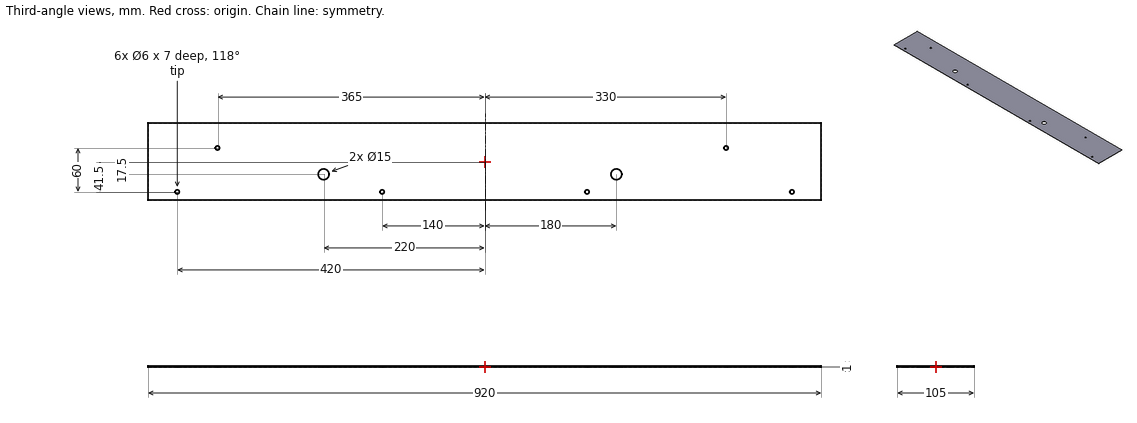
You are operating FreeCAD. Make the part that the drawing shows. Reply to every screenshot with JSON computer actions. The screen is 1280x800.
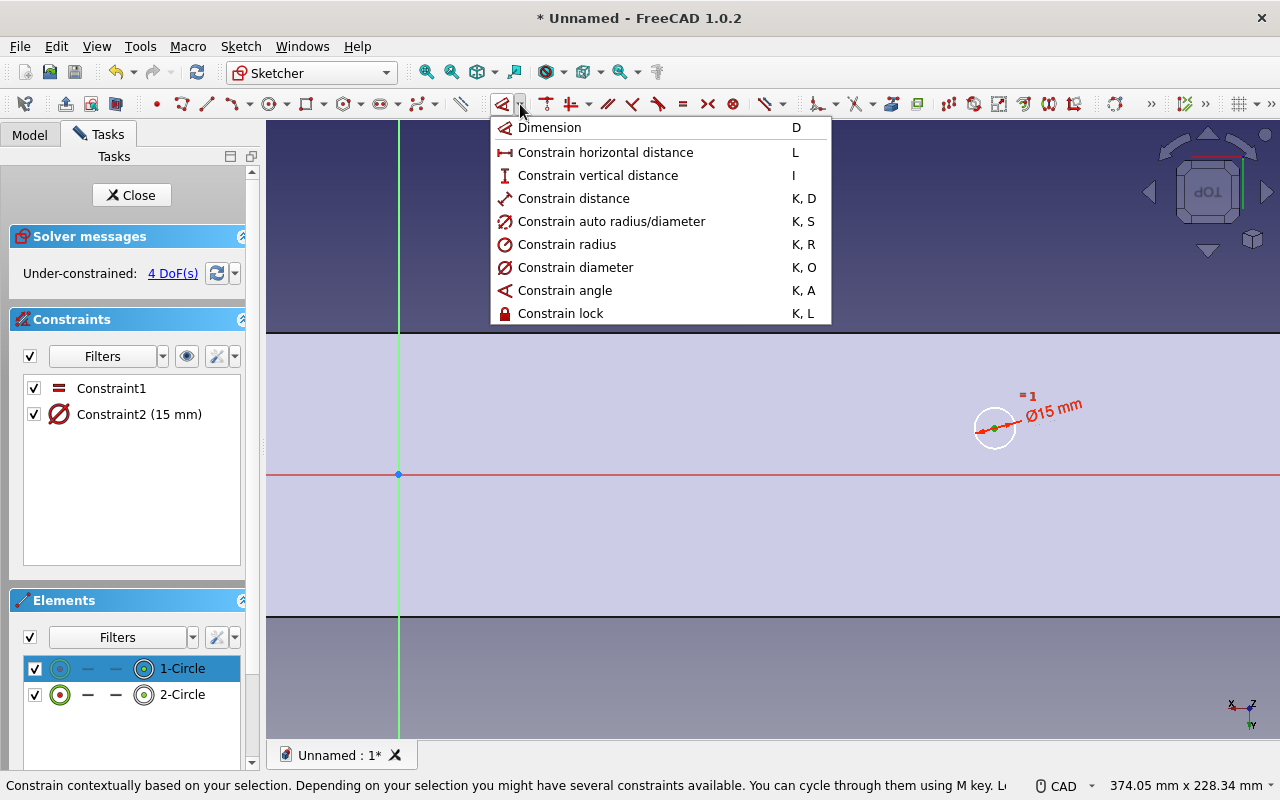
{"action": "left_click", "coordinate": [661, 152]}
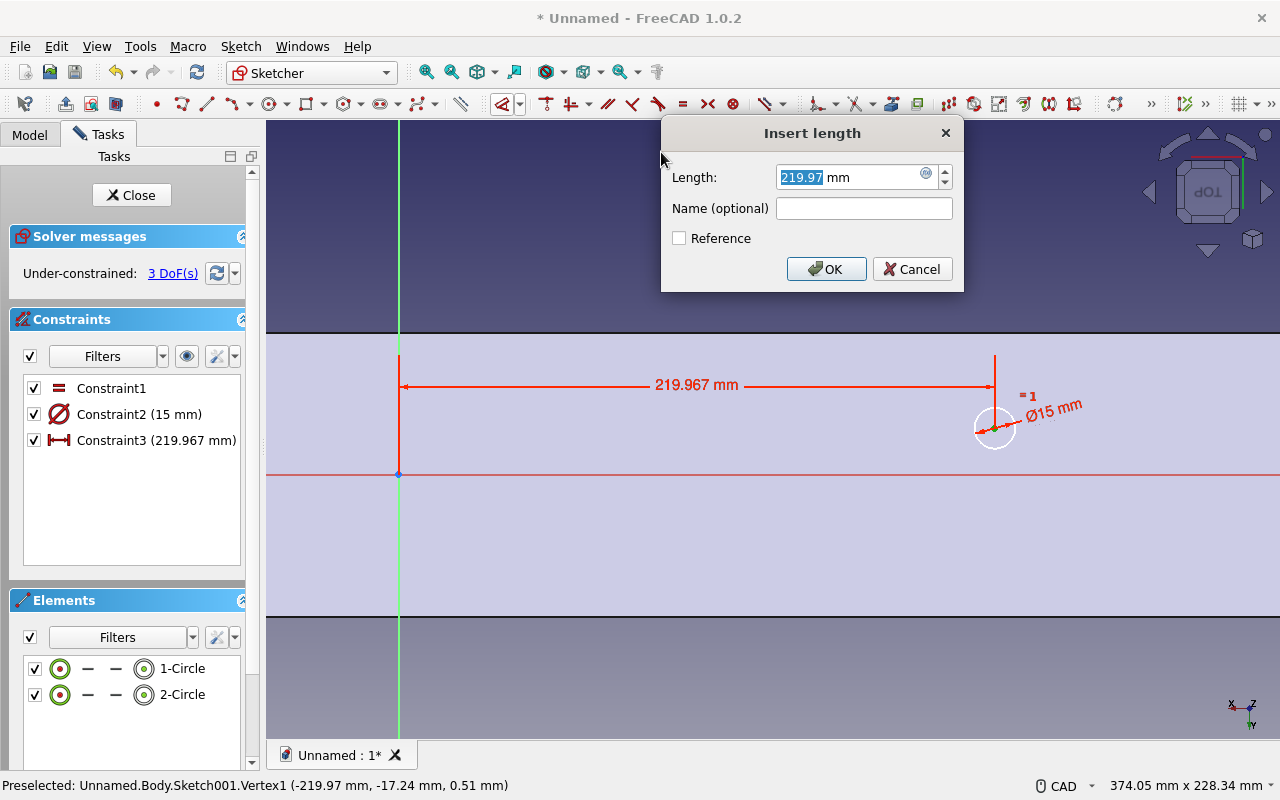
{"action": "type", "text": "220"}
{"action": "key", "text": "Return"}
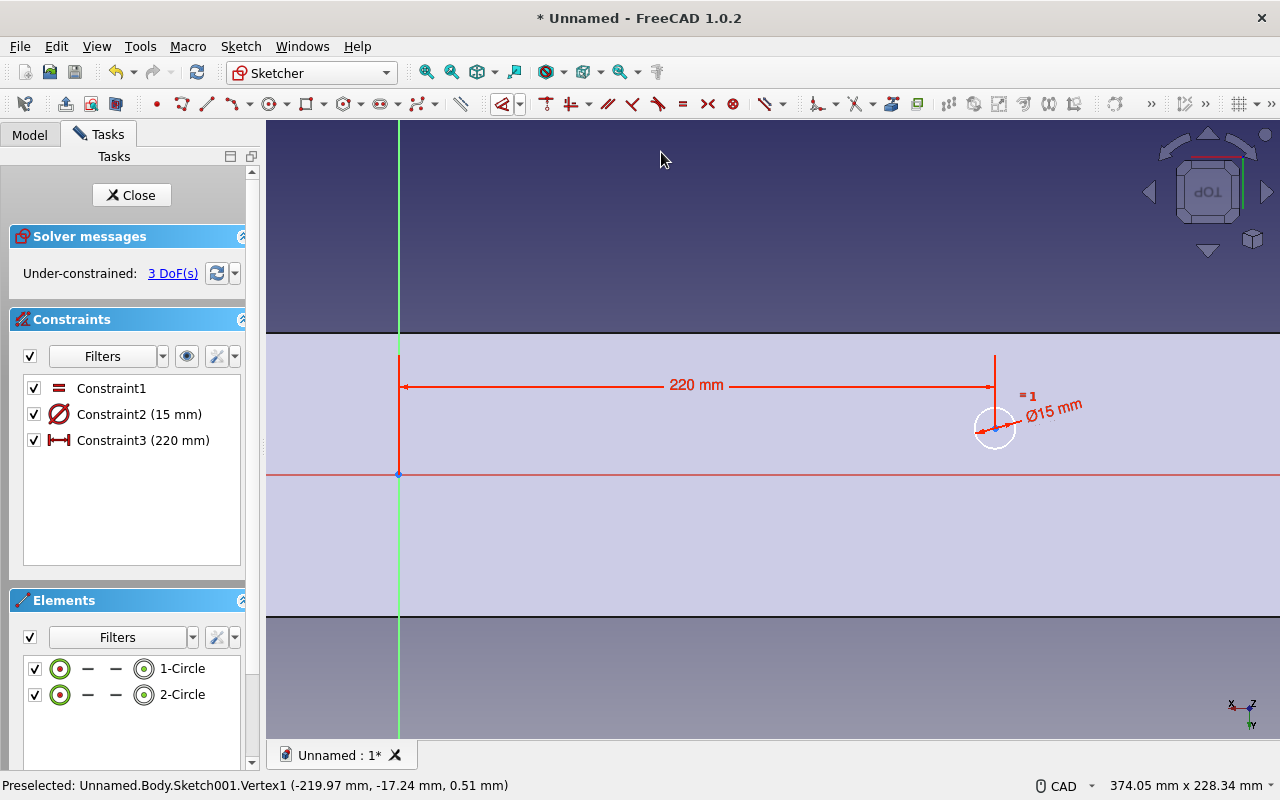
{"action": "scroll", "coordinate": [1011, 415], "scroll_direction": "down", "scroll_amount": 3}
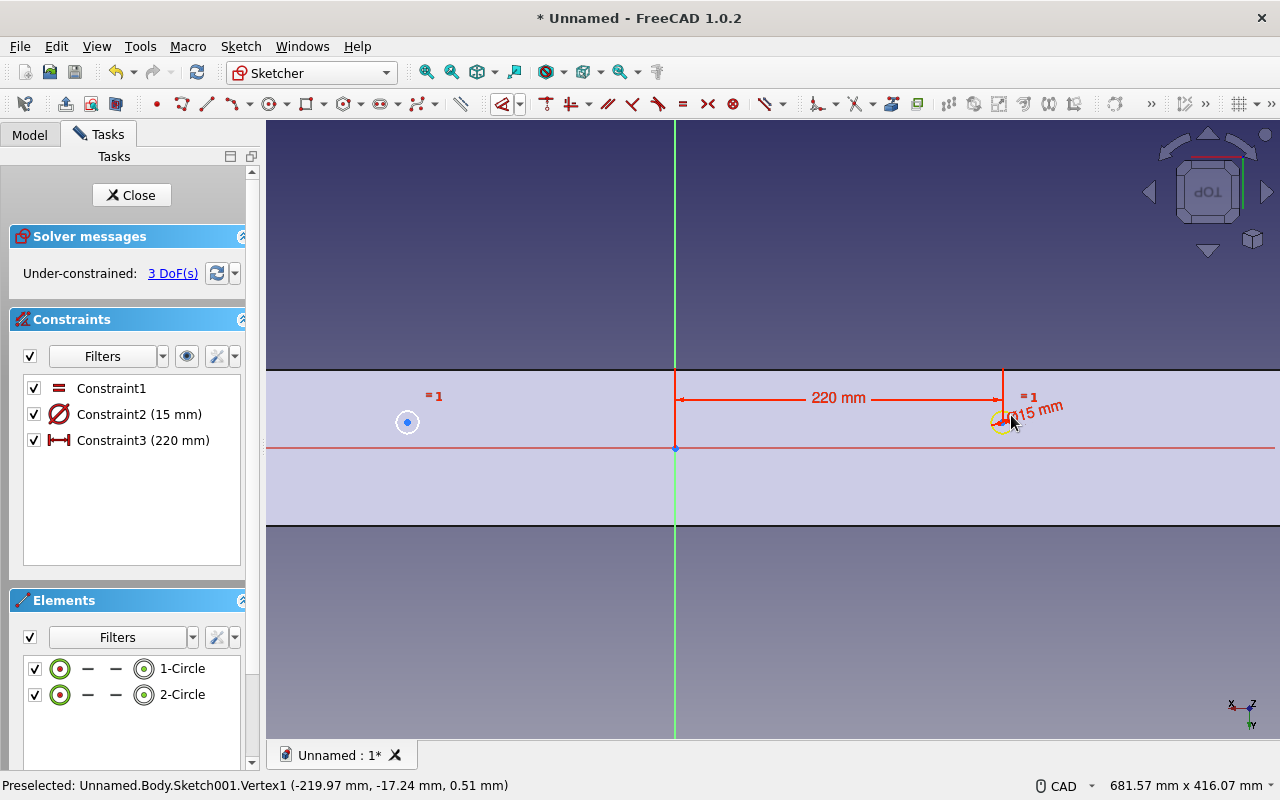
{"action": "left_click", "coordinate": [408, 422]}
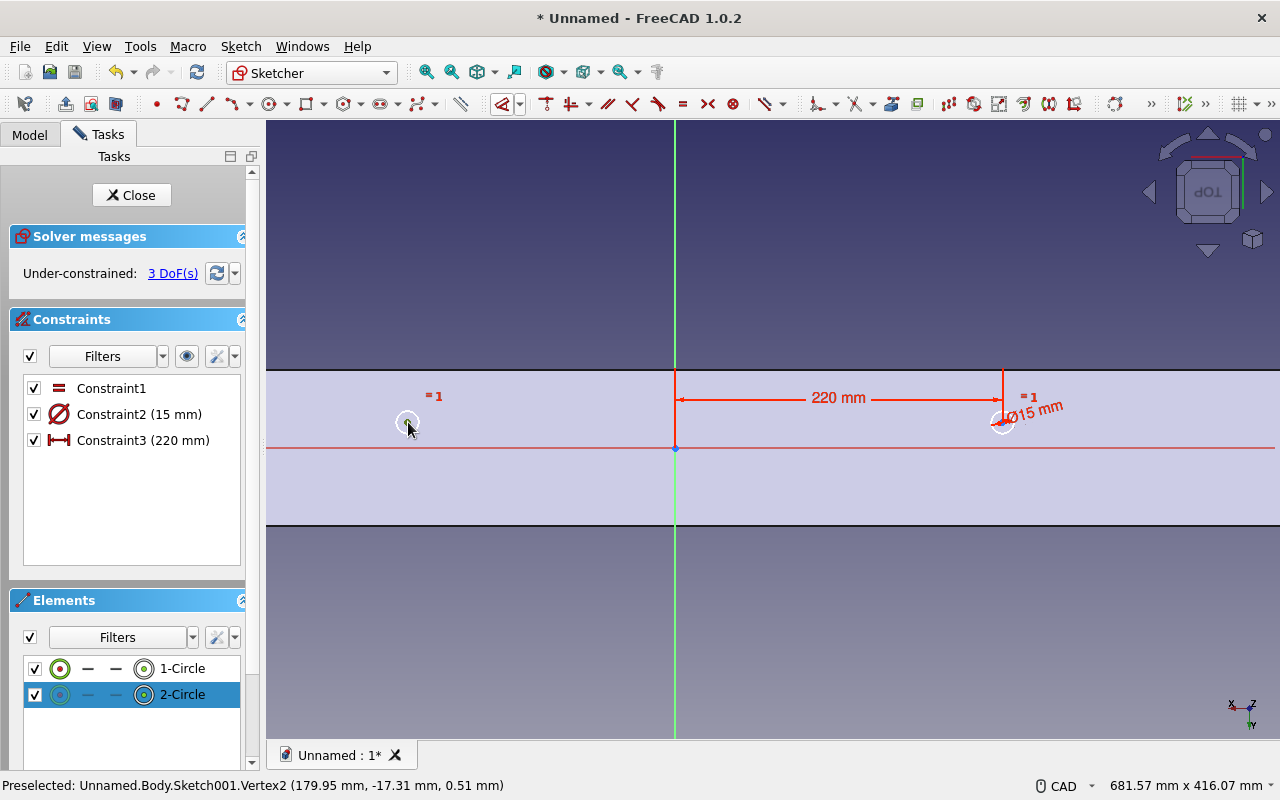
{"action": "left_click", "coordinate": [520, 104]}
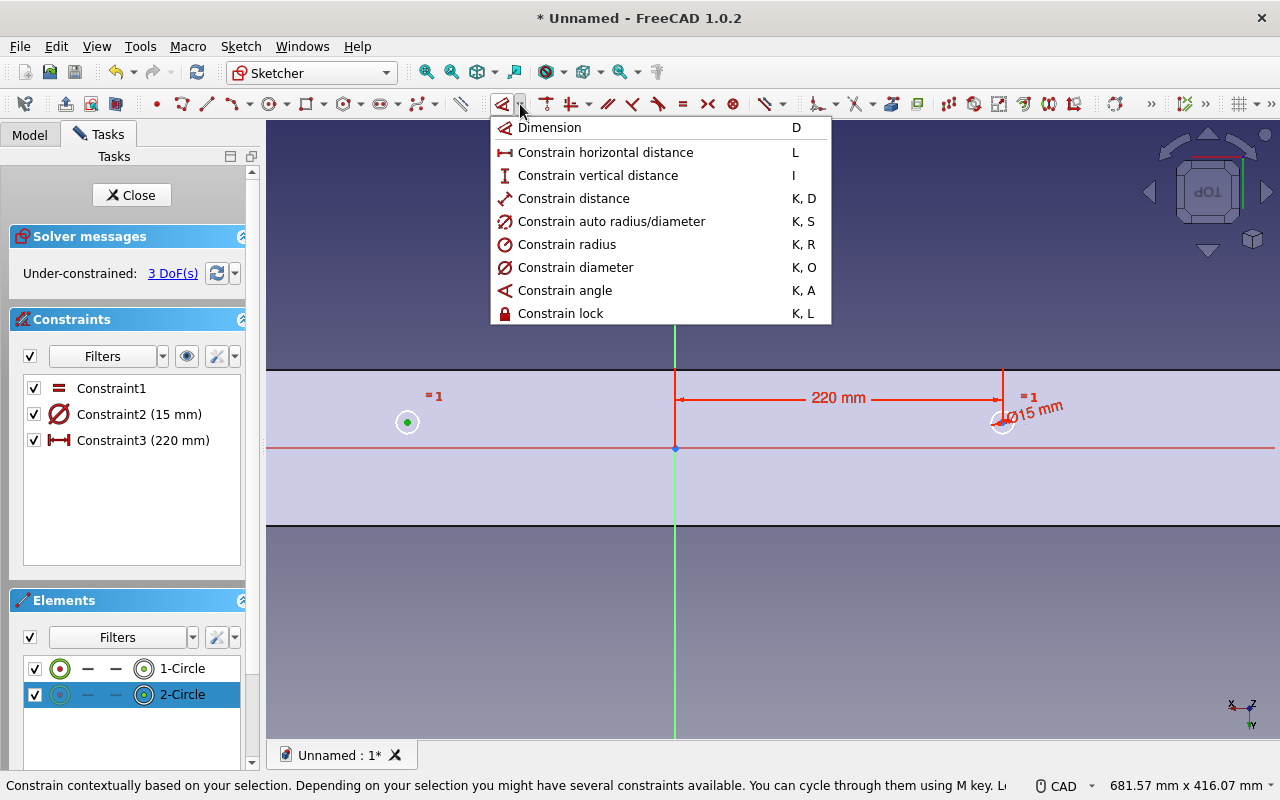
{"action": "left_click", "coordinate": [661, 152]}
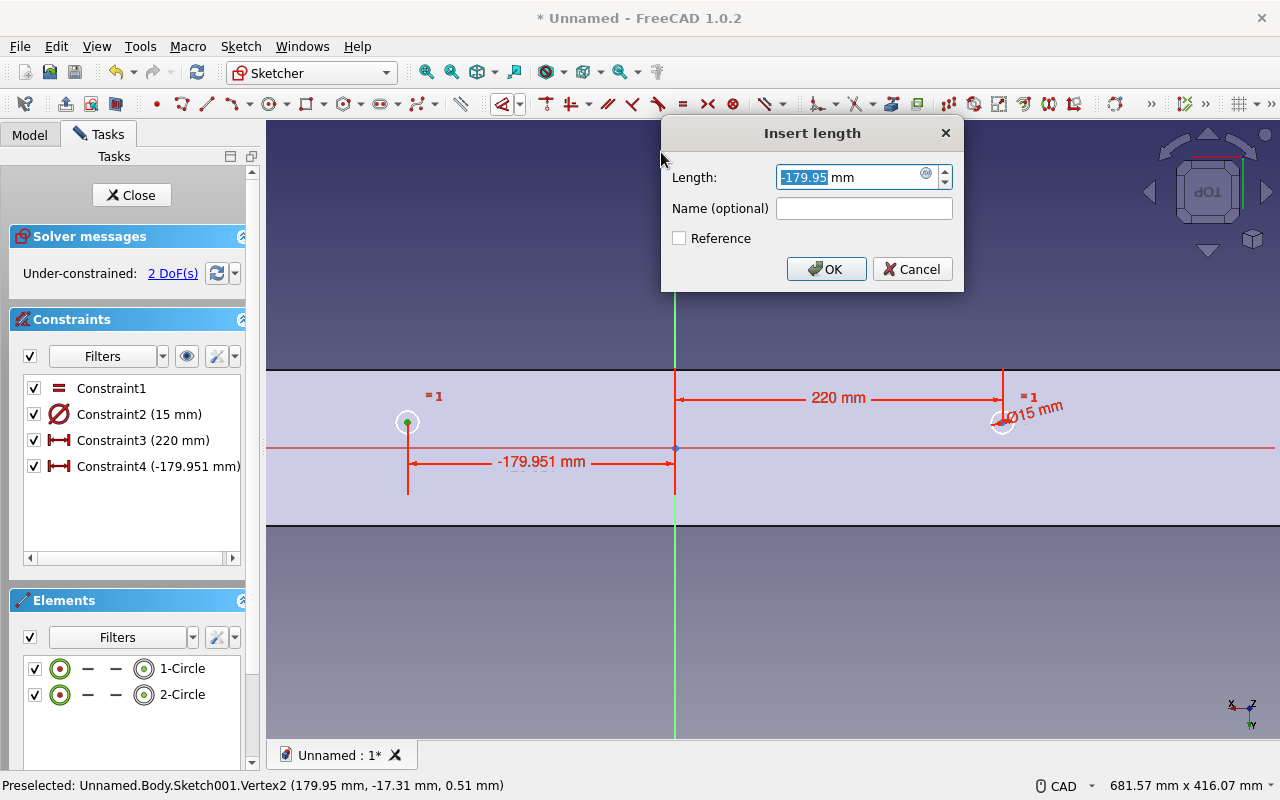
{"action": "type", "text": "-180"}
{"action": "key", "text": "Return"}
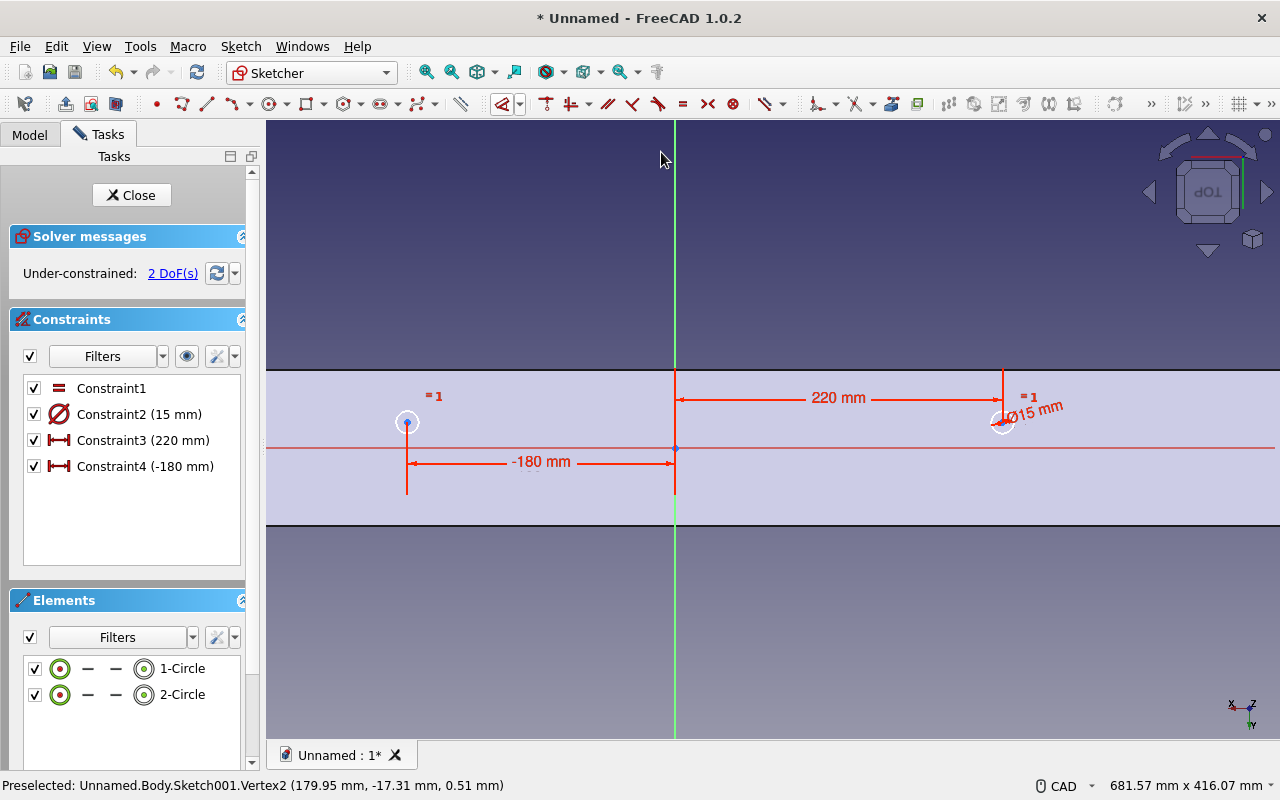
{"action": "scroll", "coordinate": [1003, 422], "scroll_direction": "up", "scroll_amount": 3}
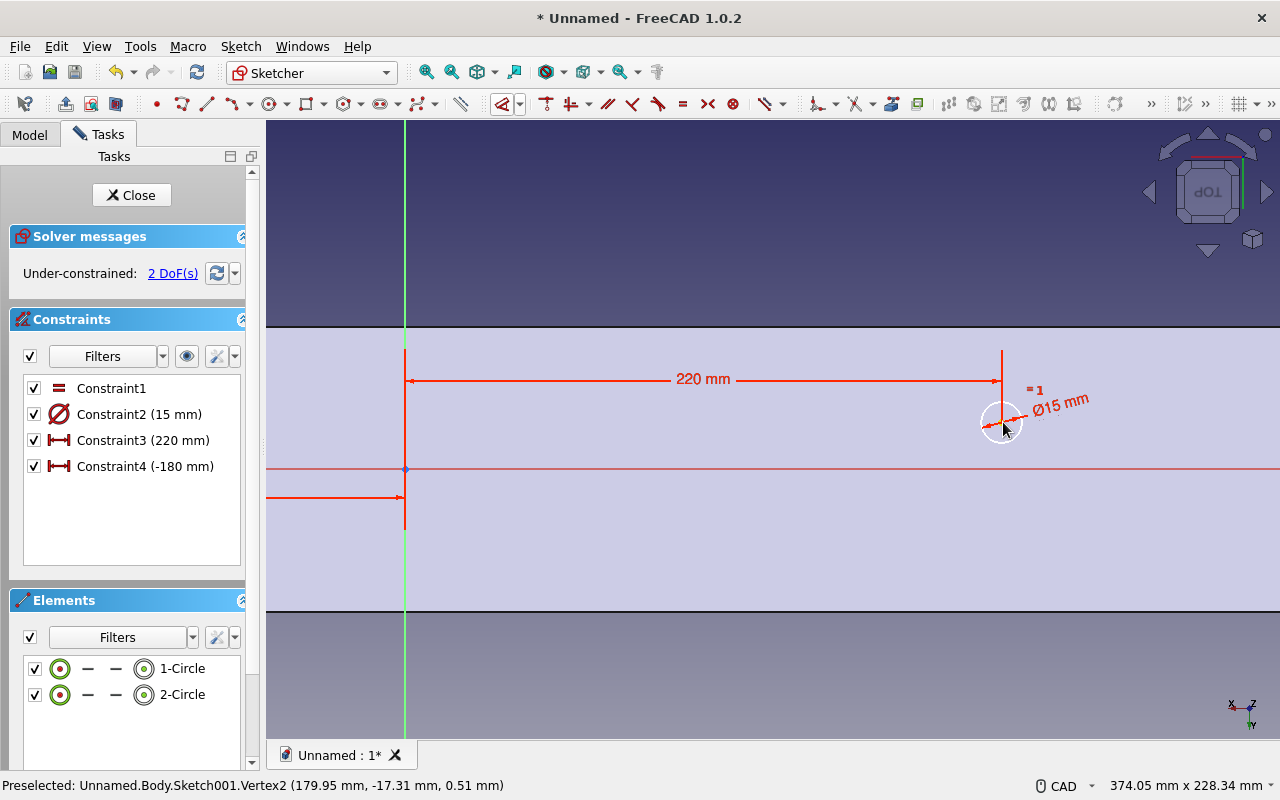
{"action": "left_click", "coordinate": [1002, 422]}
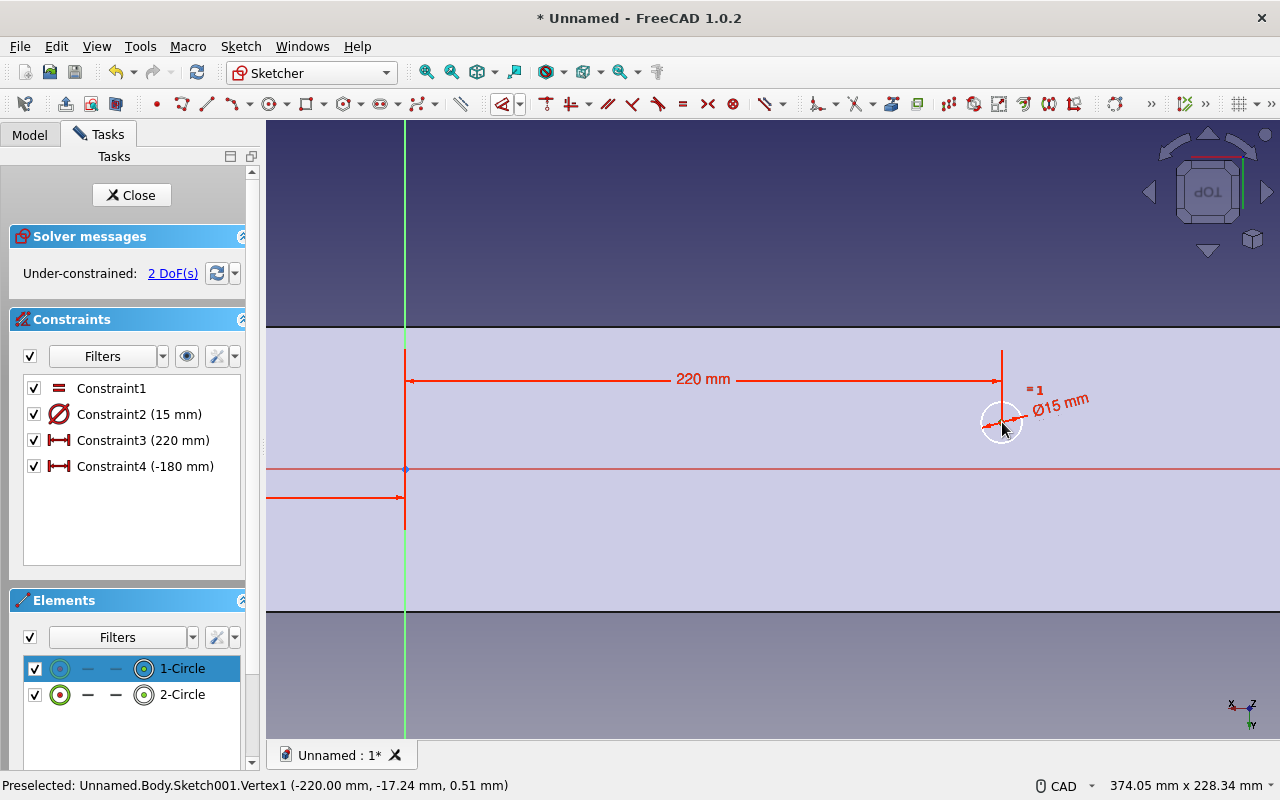
{"action": "left_click", "coordinate": [520, 104]}